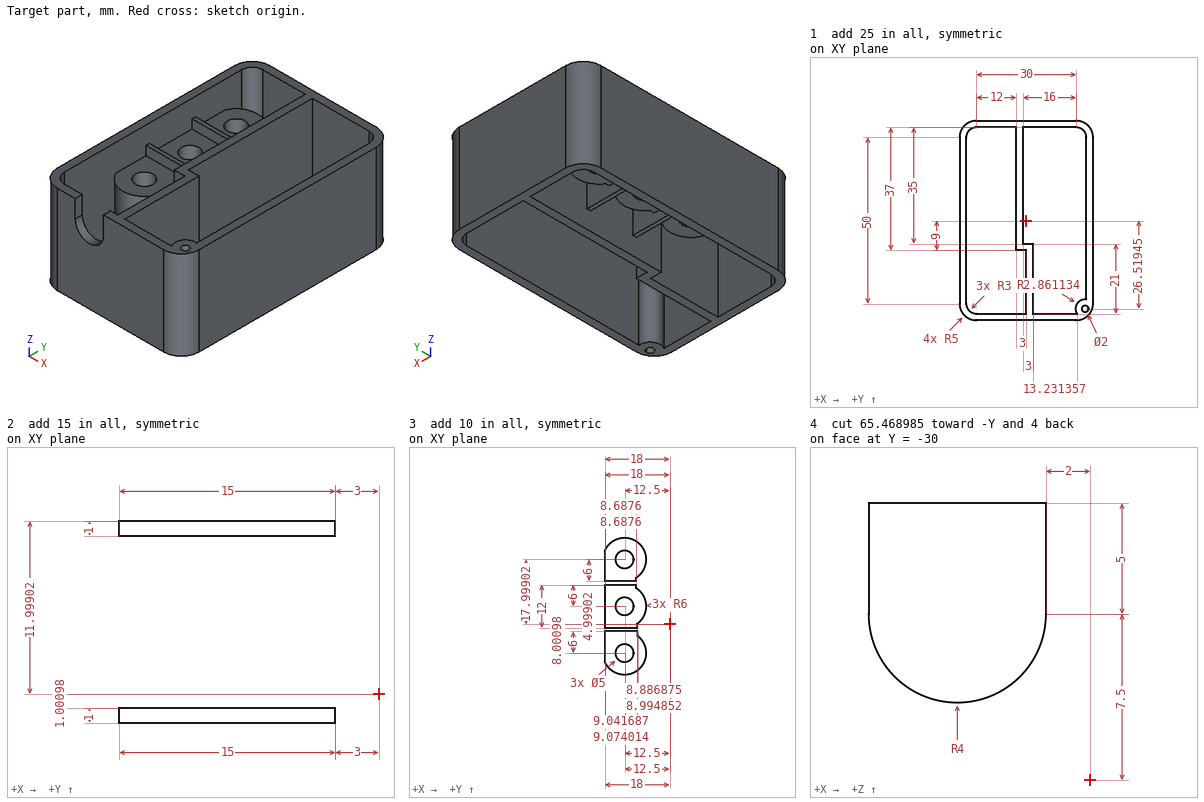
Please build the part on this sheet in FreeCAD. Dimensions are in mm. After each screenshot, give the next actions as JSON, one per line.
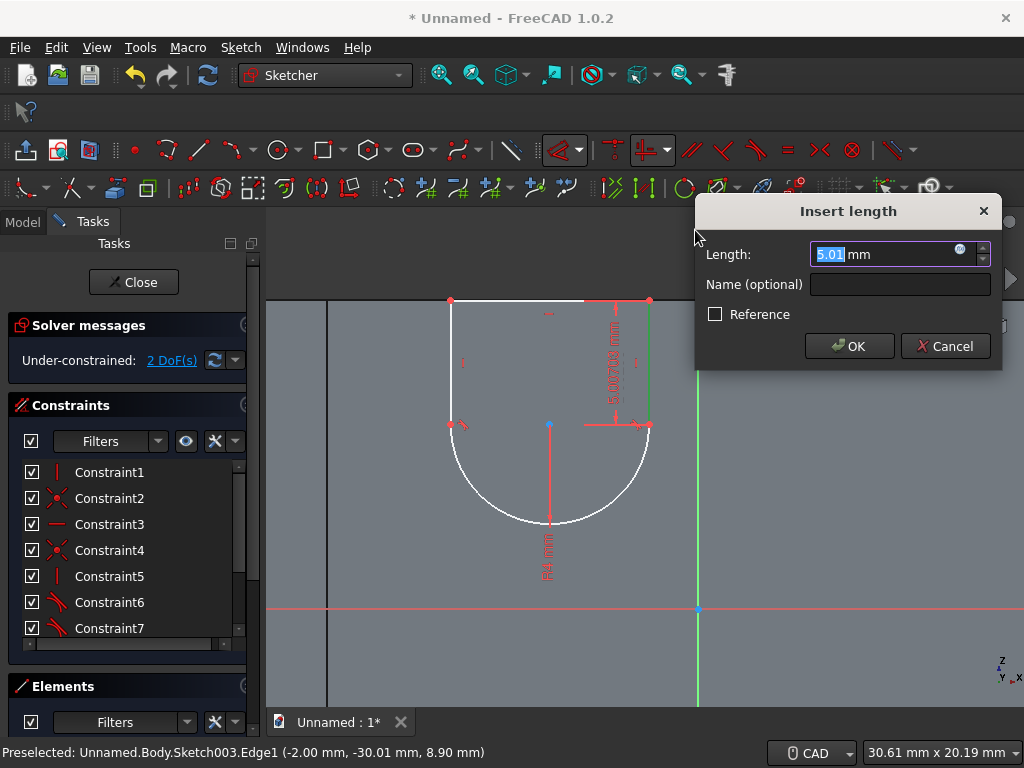
{"action": "type", "text": "5"}
{"action": "key", "text": "Return"}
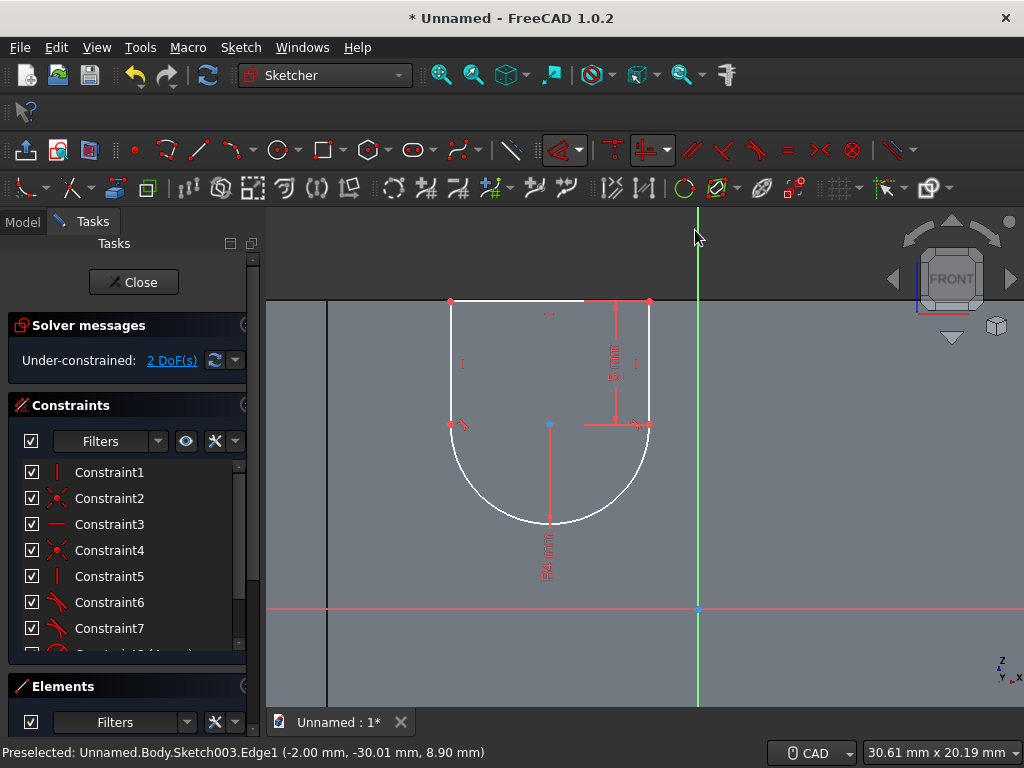
{"action": "left_click", "coordinate": [649, 425]}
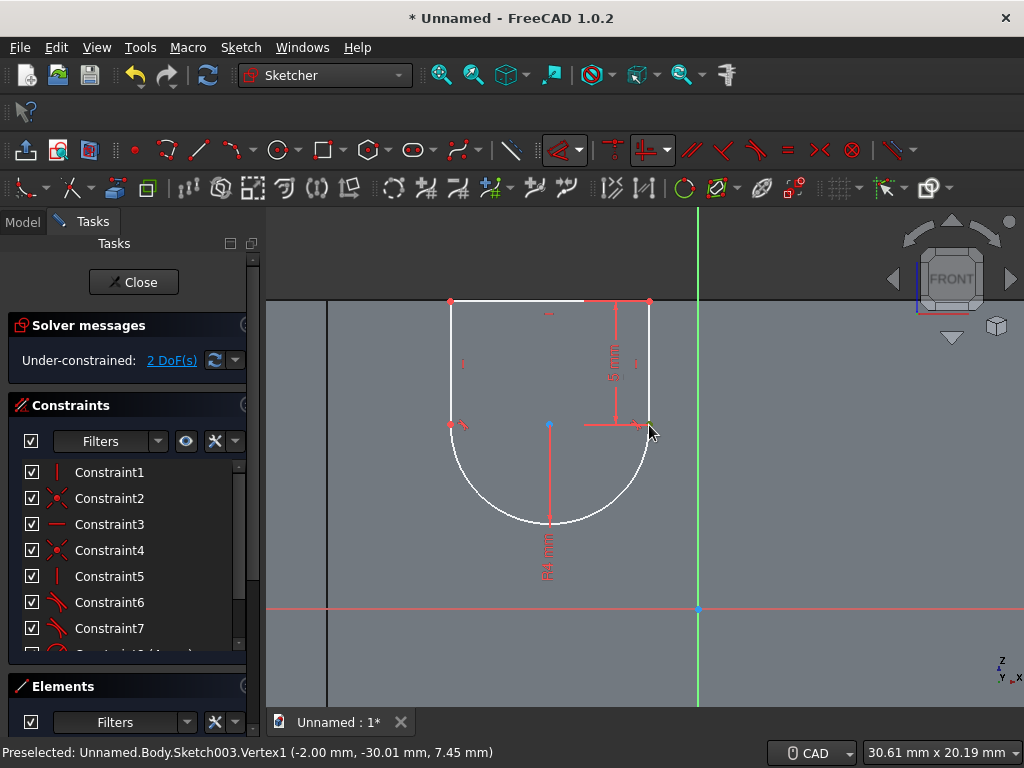
{"action": "key", "text": "l"}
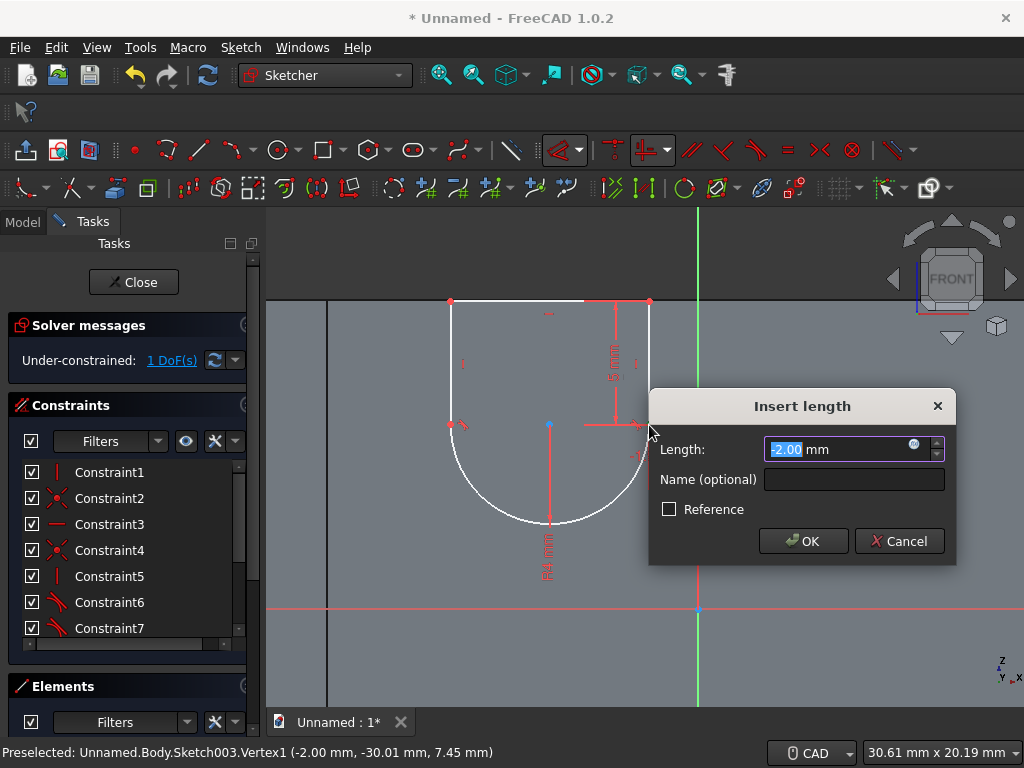
{"action": "type", "text": "-2"}
{"action": "key", "text": "Return"}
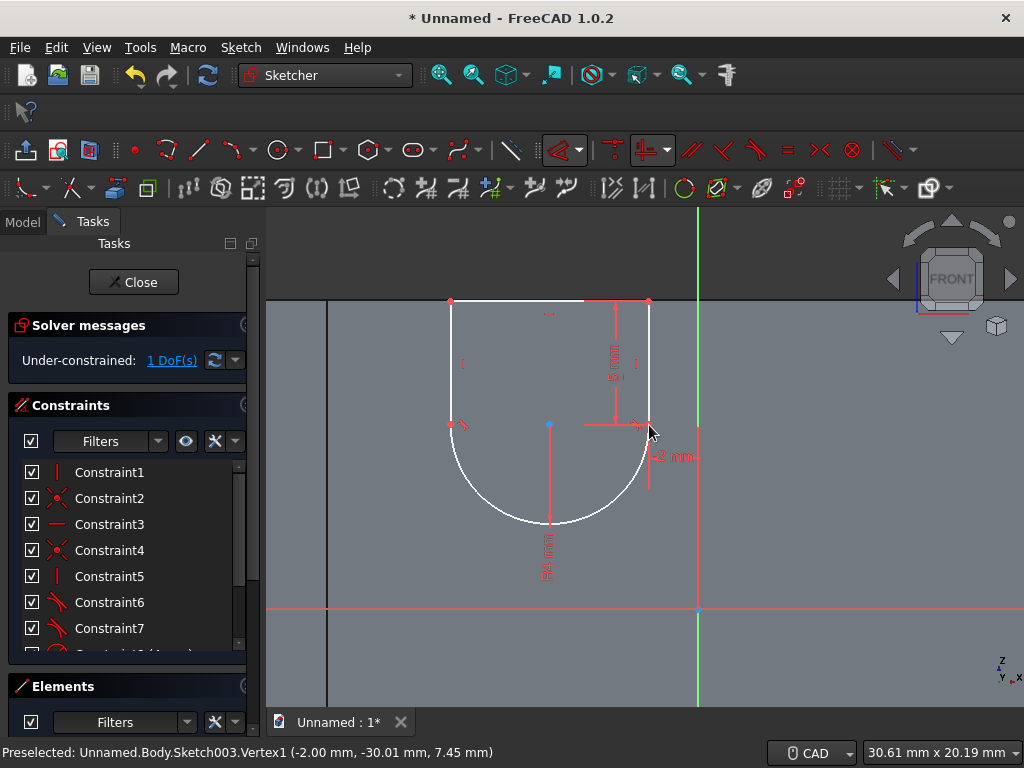
{"action": "left_click", "coordinate": [649, 425]}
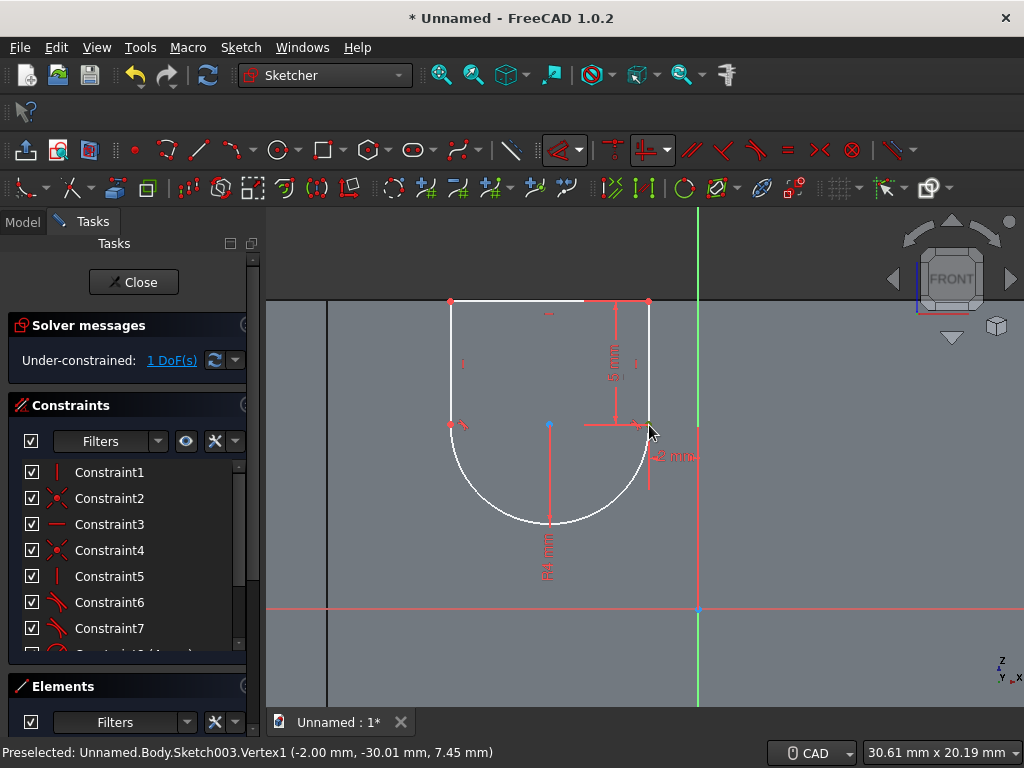
{"action": "key", "text": "i"}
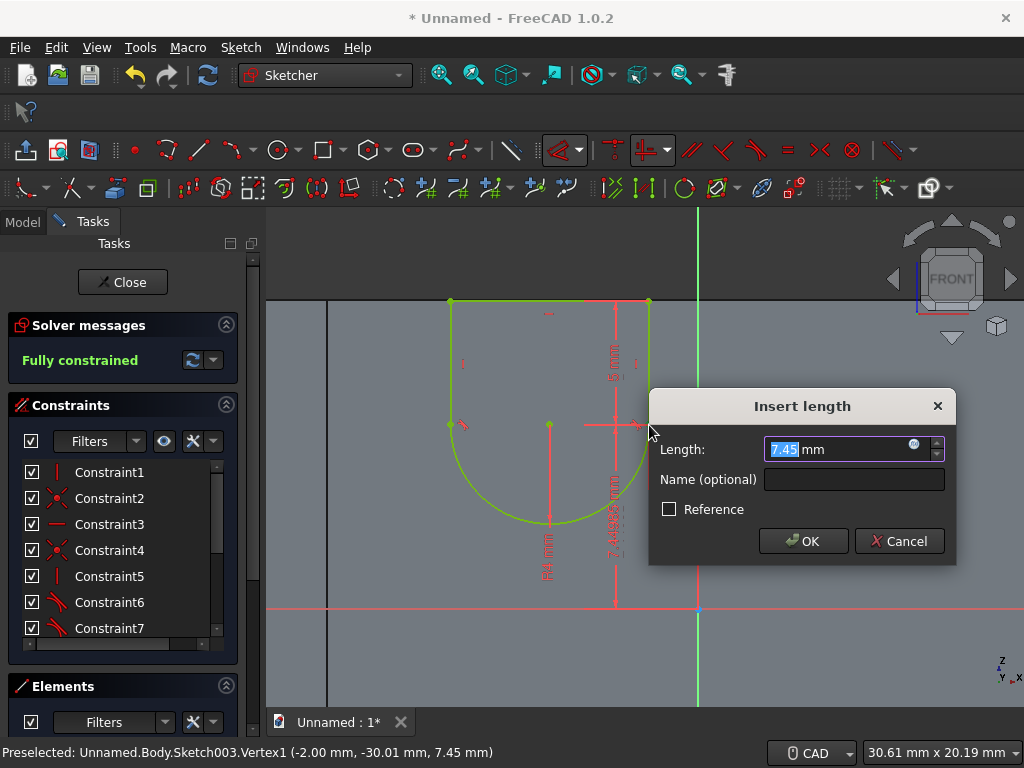
{"action": "type", "text": "7.5"}
{"action": "key", "text": "Return"}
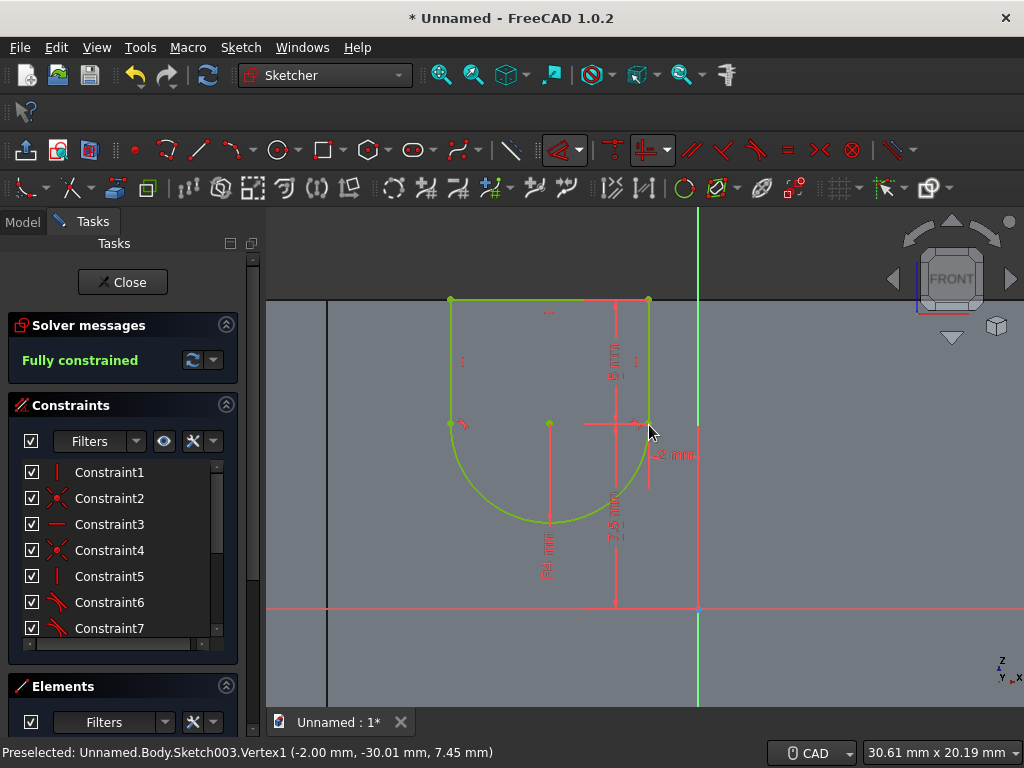
{"action": "left_click", "coordinate": [123, 282]}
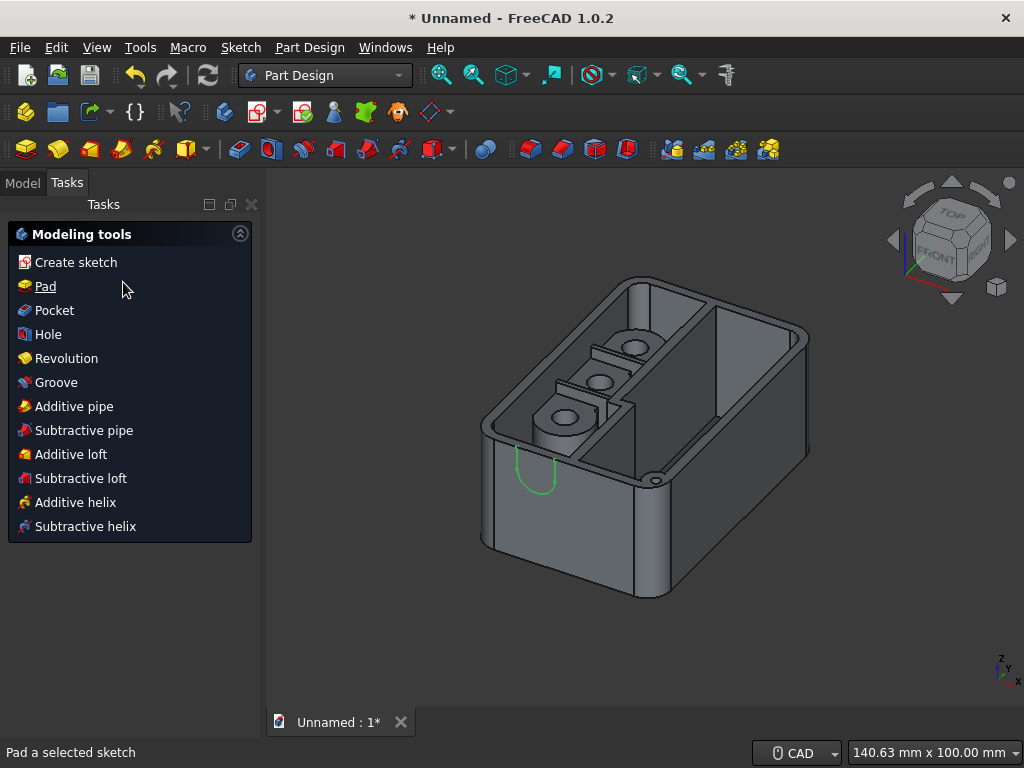
{"action": "left_click", "coordinate": [240, 150]}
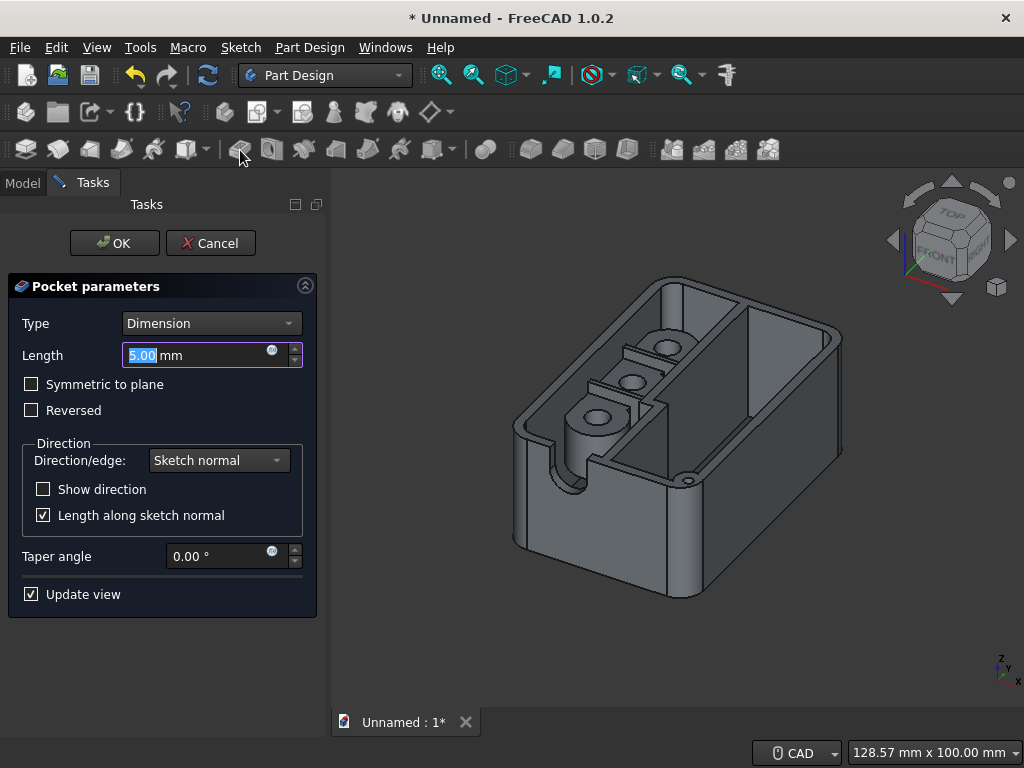
{"action": "left_click", "coordinate": [212, 324]}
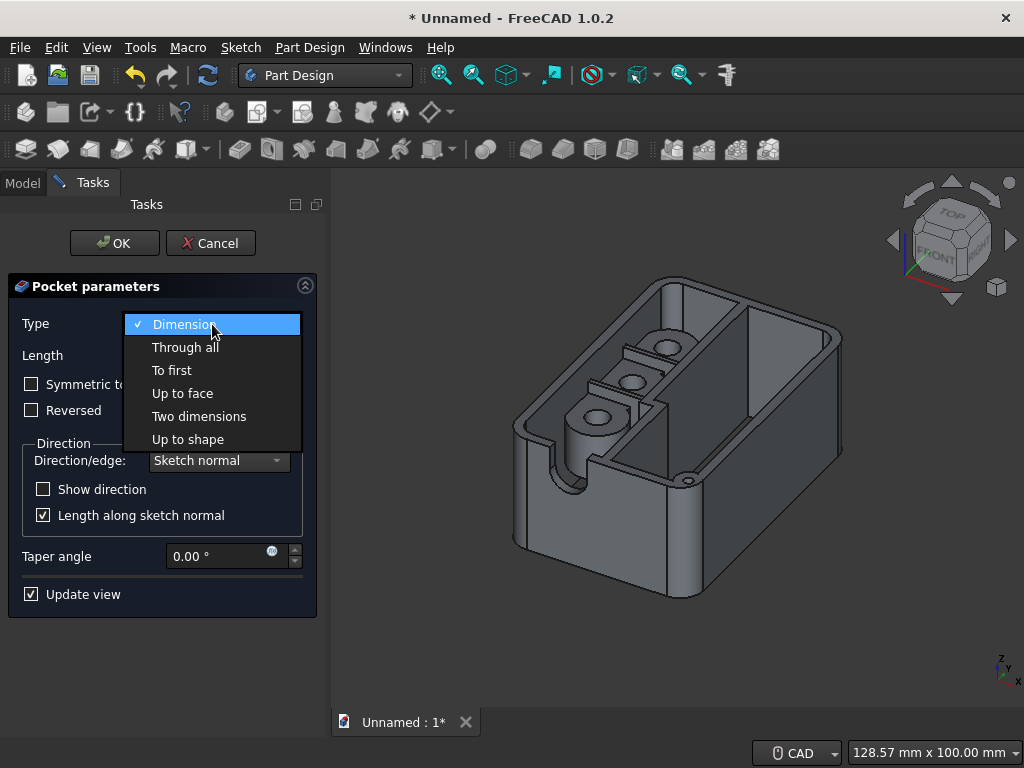
{"action": "left_click", "coordinate": [212, 416]}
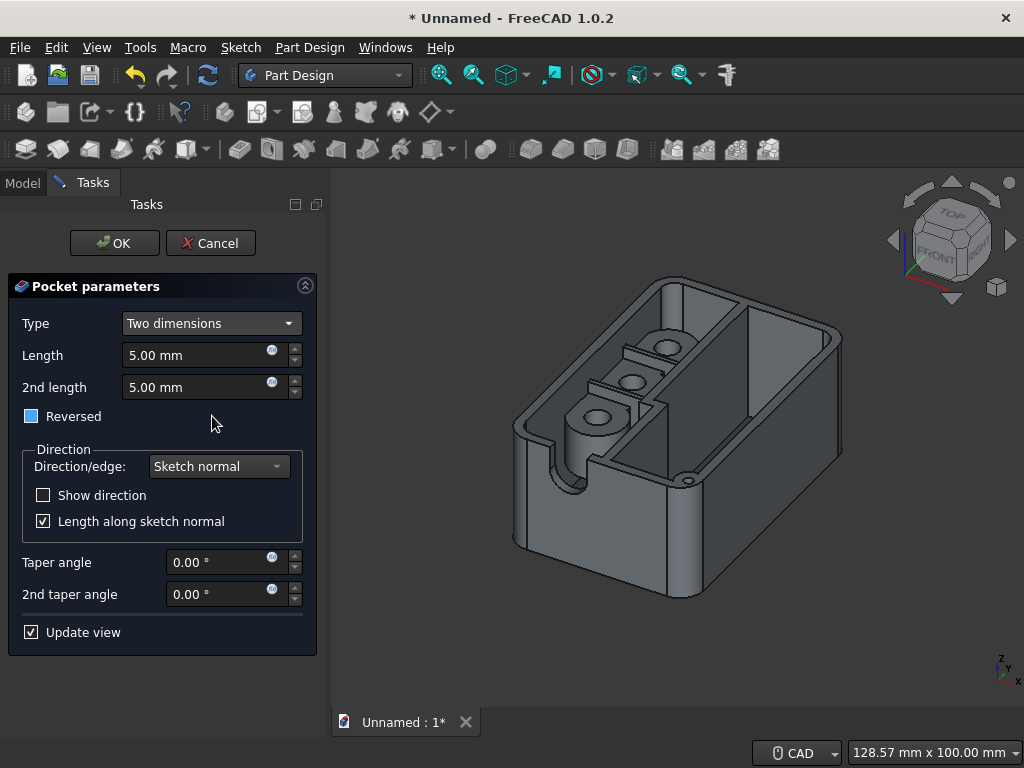
{"action": "triple_click", "coordinate": [204, 355]}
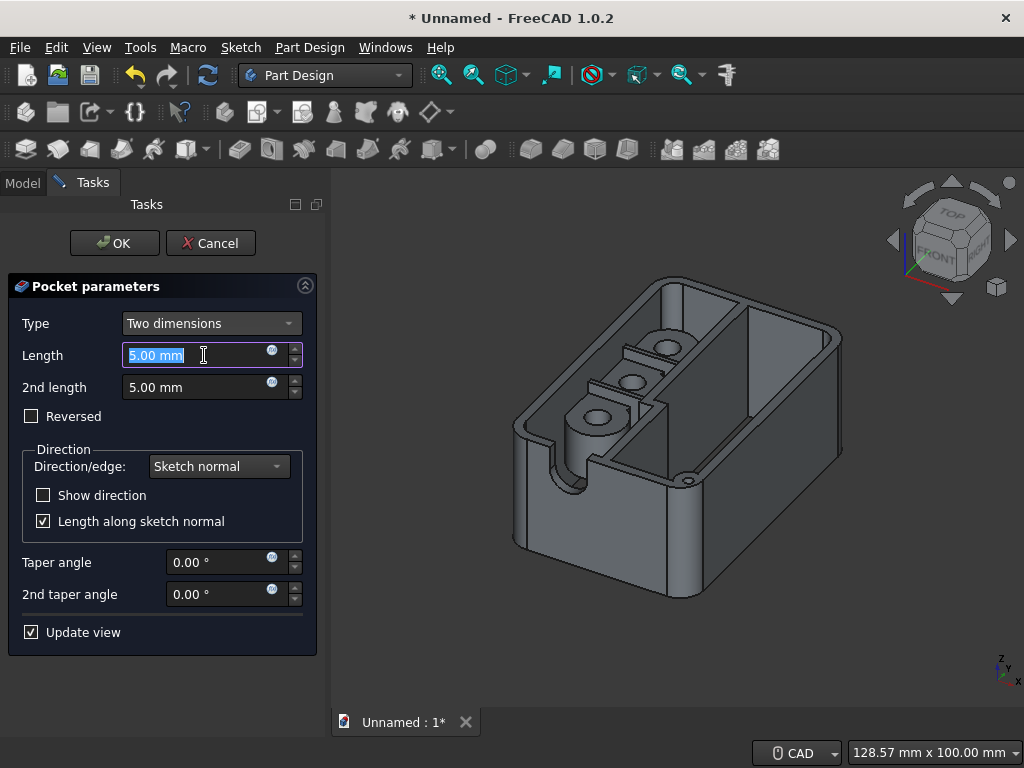
{"action": "type", "text": "65.468985"}
{"action": "key", "text": "Tab"}